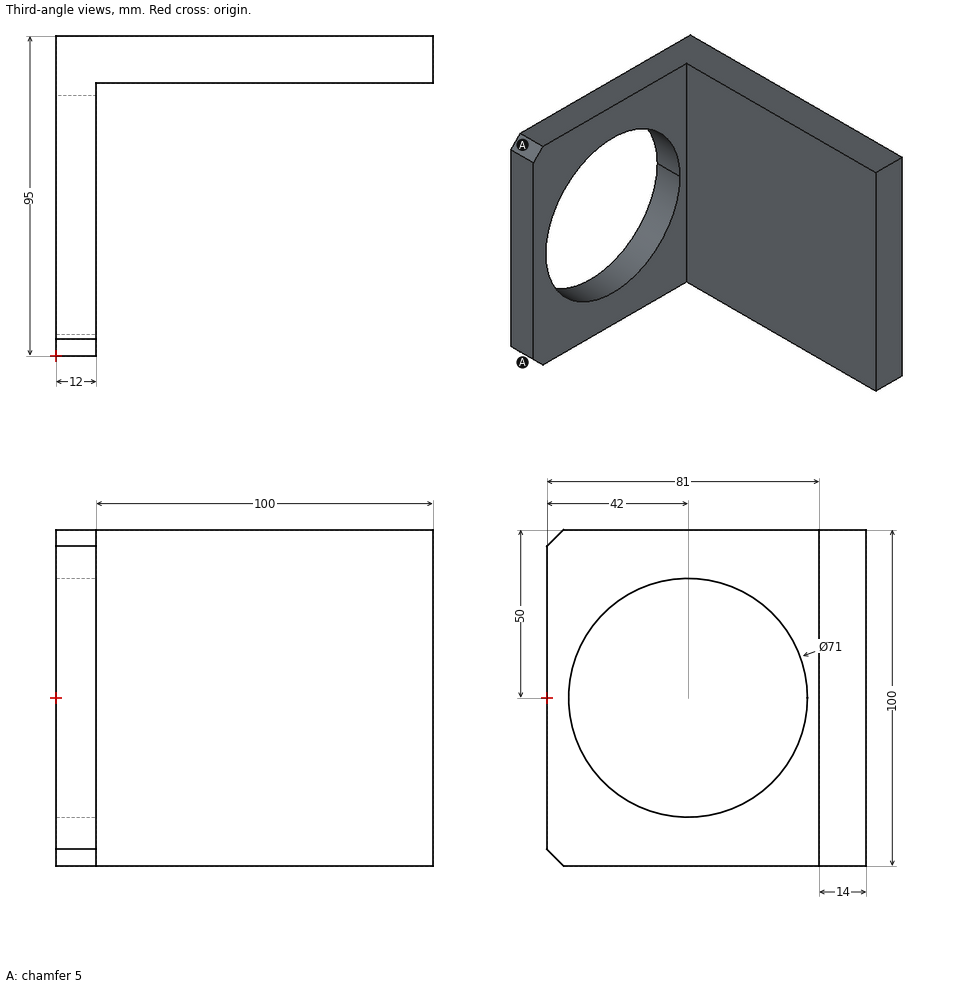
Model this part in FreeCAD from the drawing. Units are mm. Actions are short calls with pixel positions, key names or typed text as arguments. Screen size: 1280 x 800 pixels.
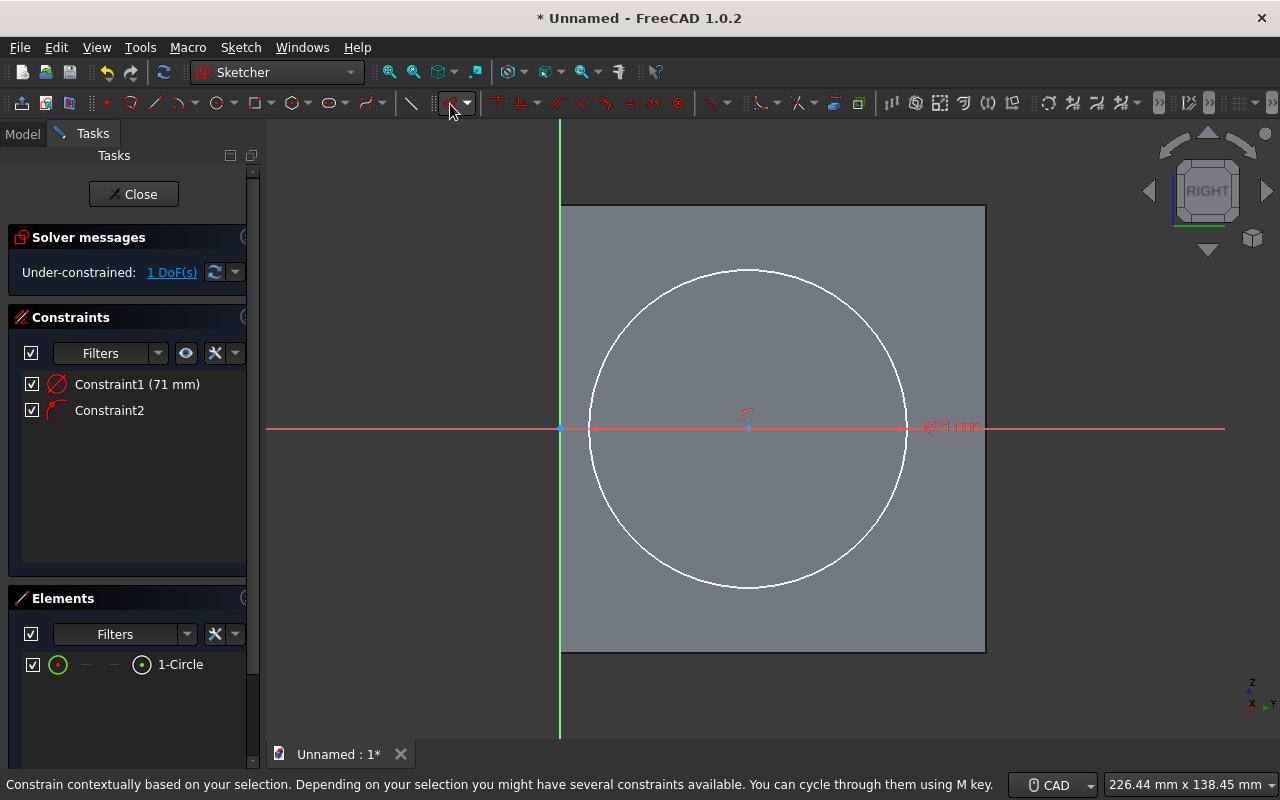
click(748, 429)
click(654, 463)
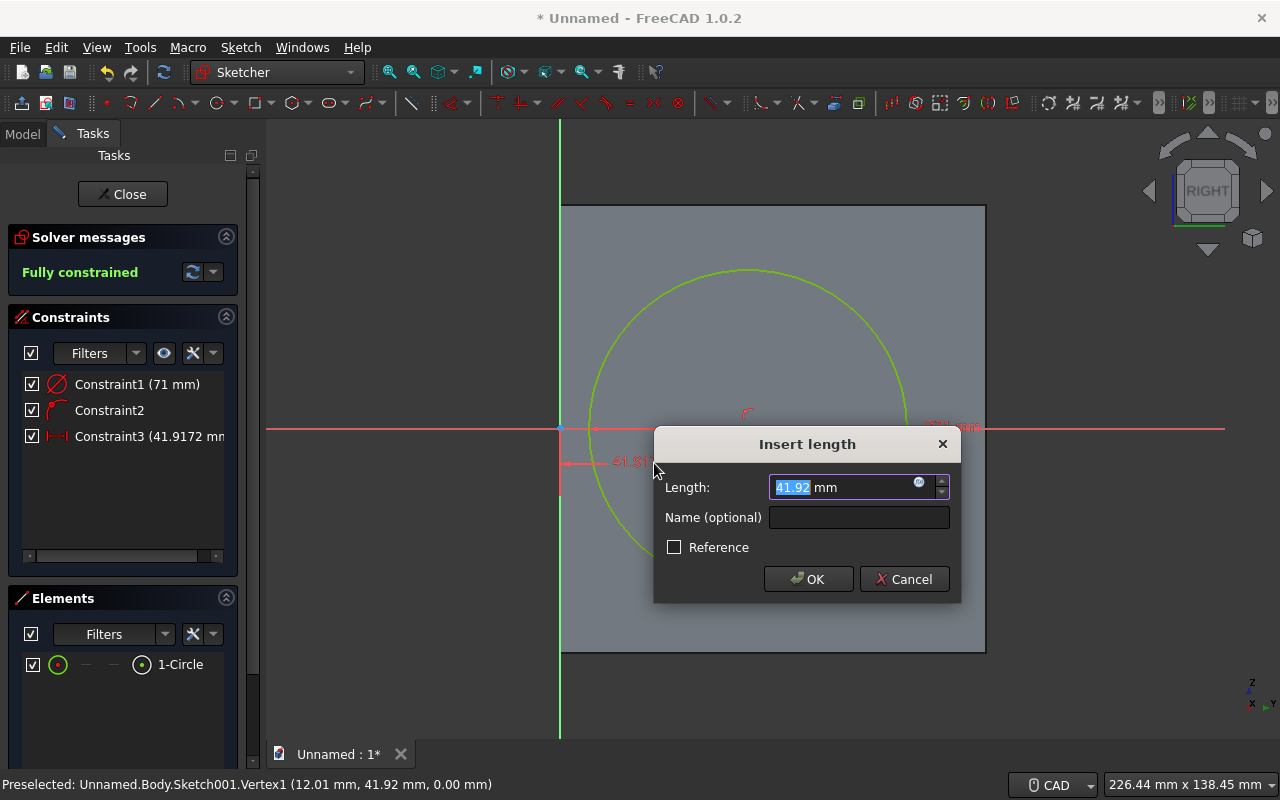
text(42)
key(Return)
key(Escape)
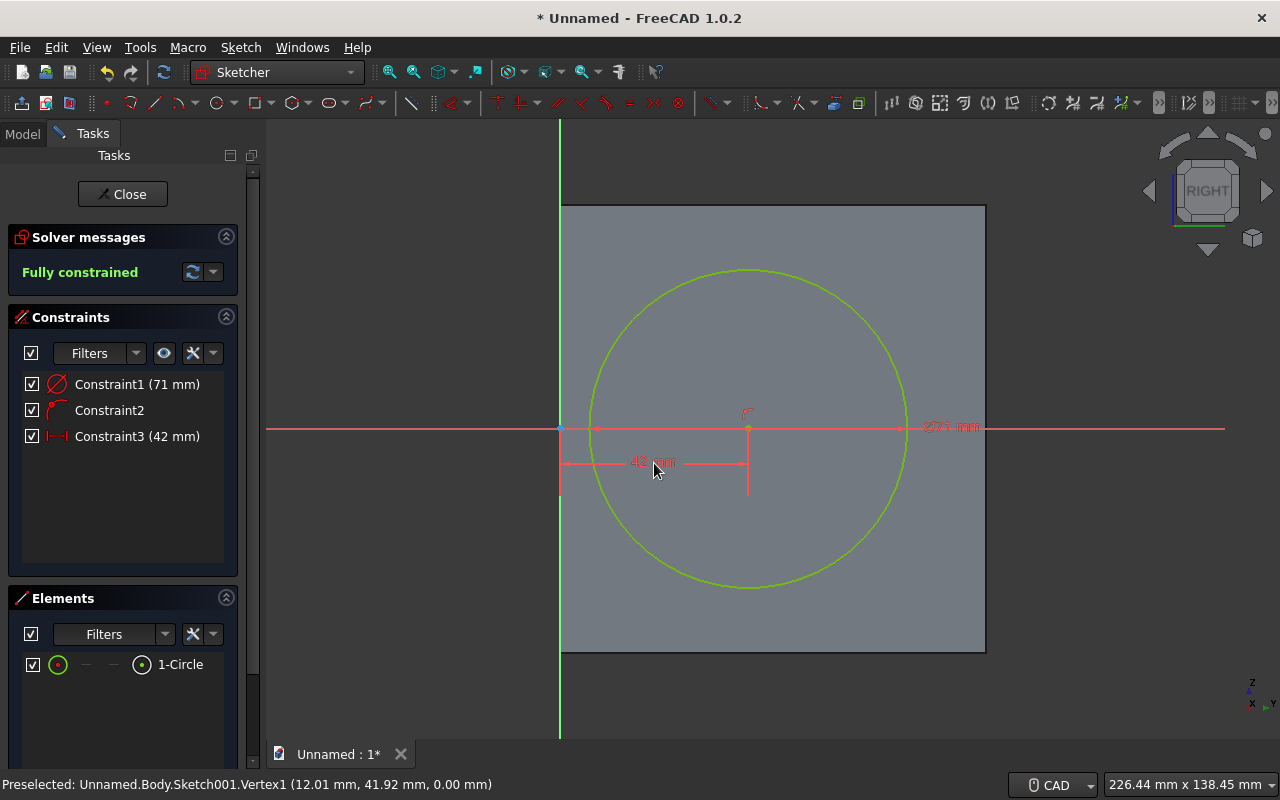
click(123, 194)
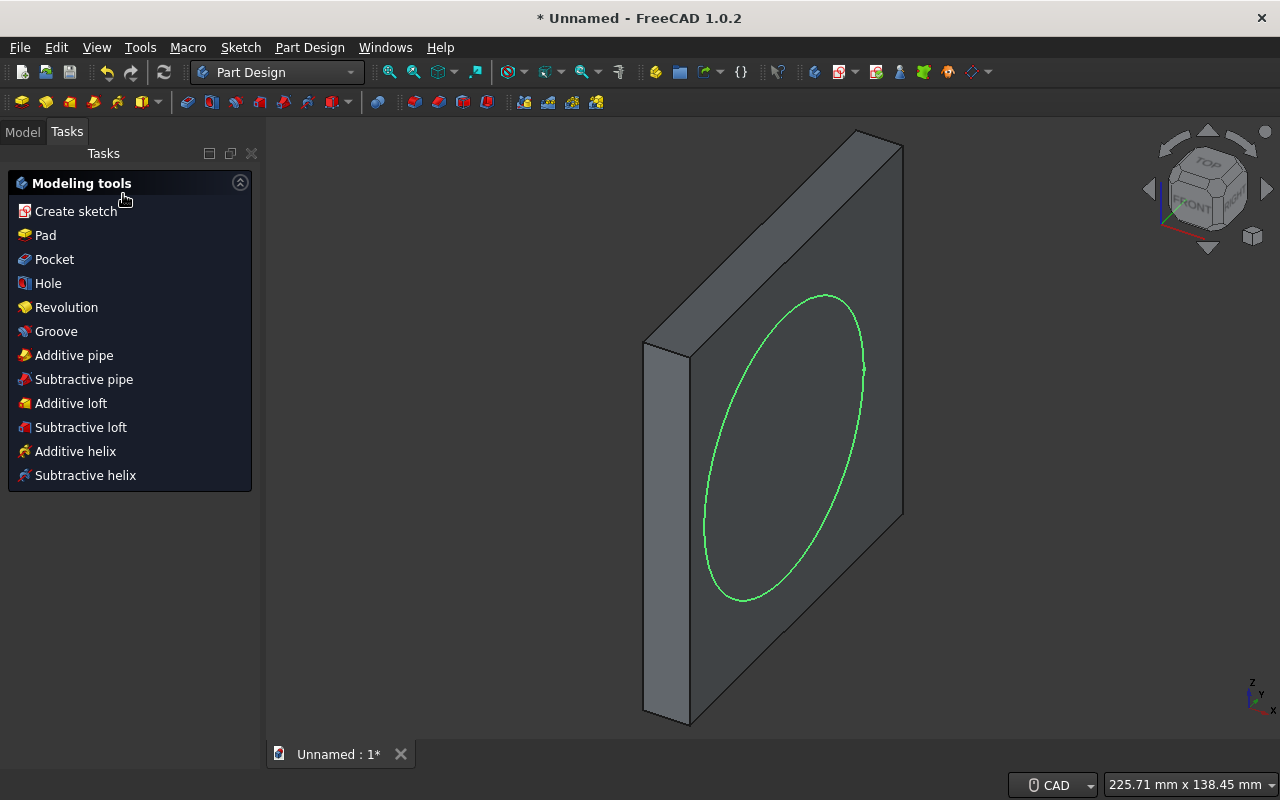
click(188, 102)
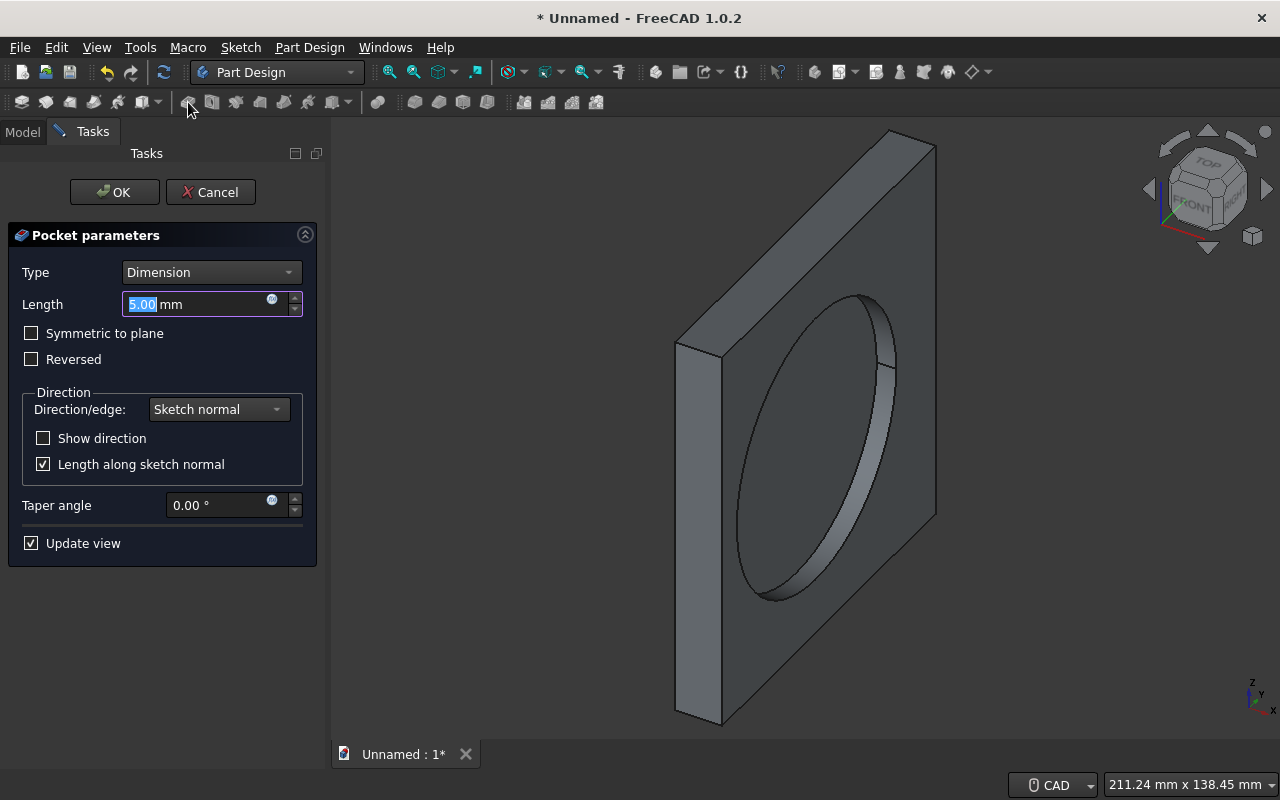
click(212, 272)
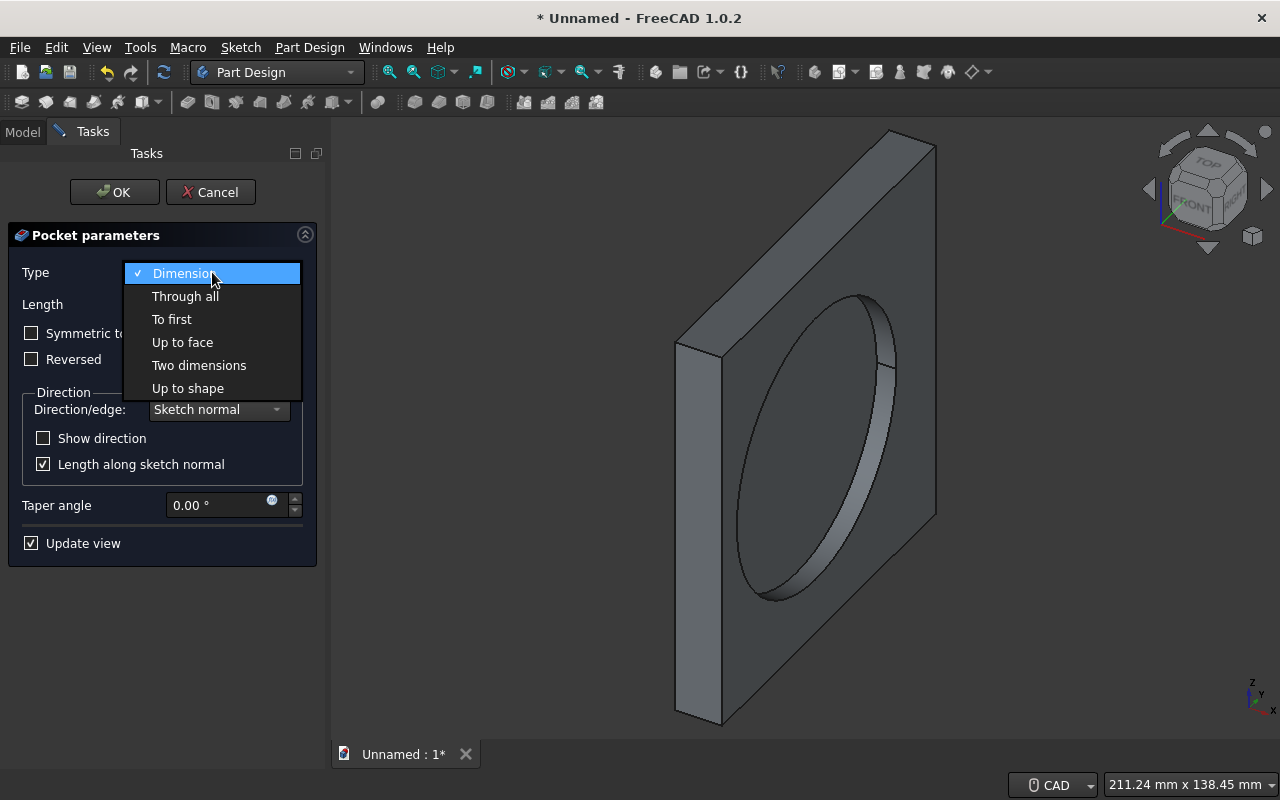
click(212, 320)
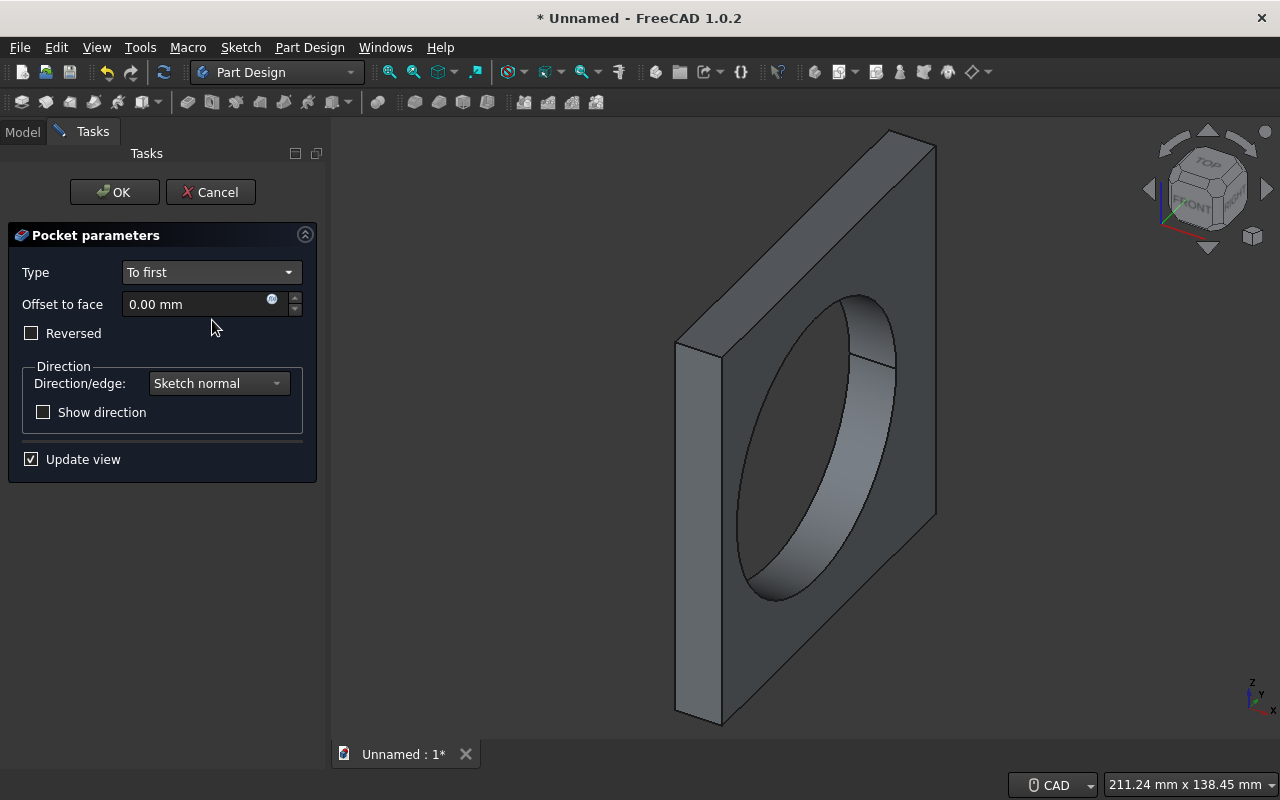
click(115, 192)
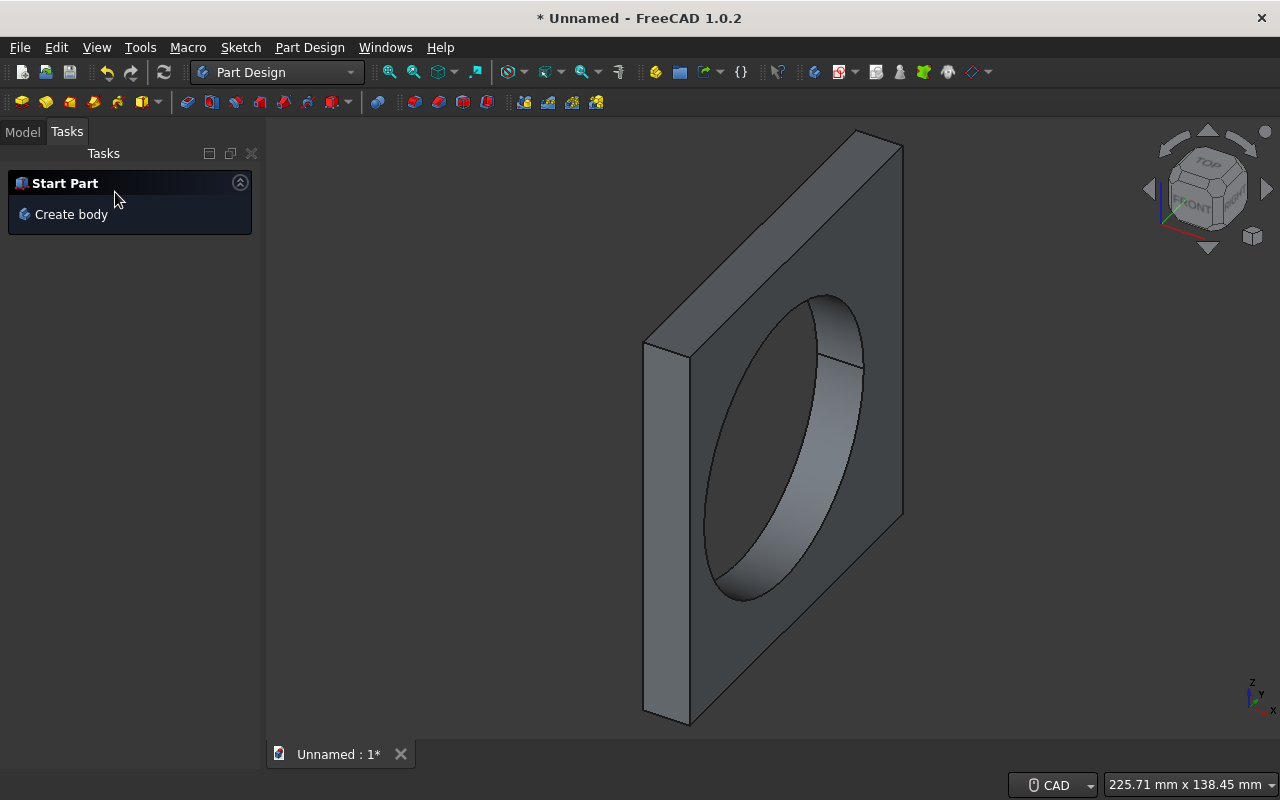
click(857, 269)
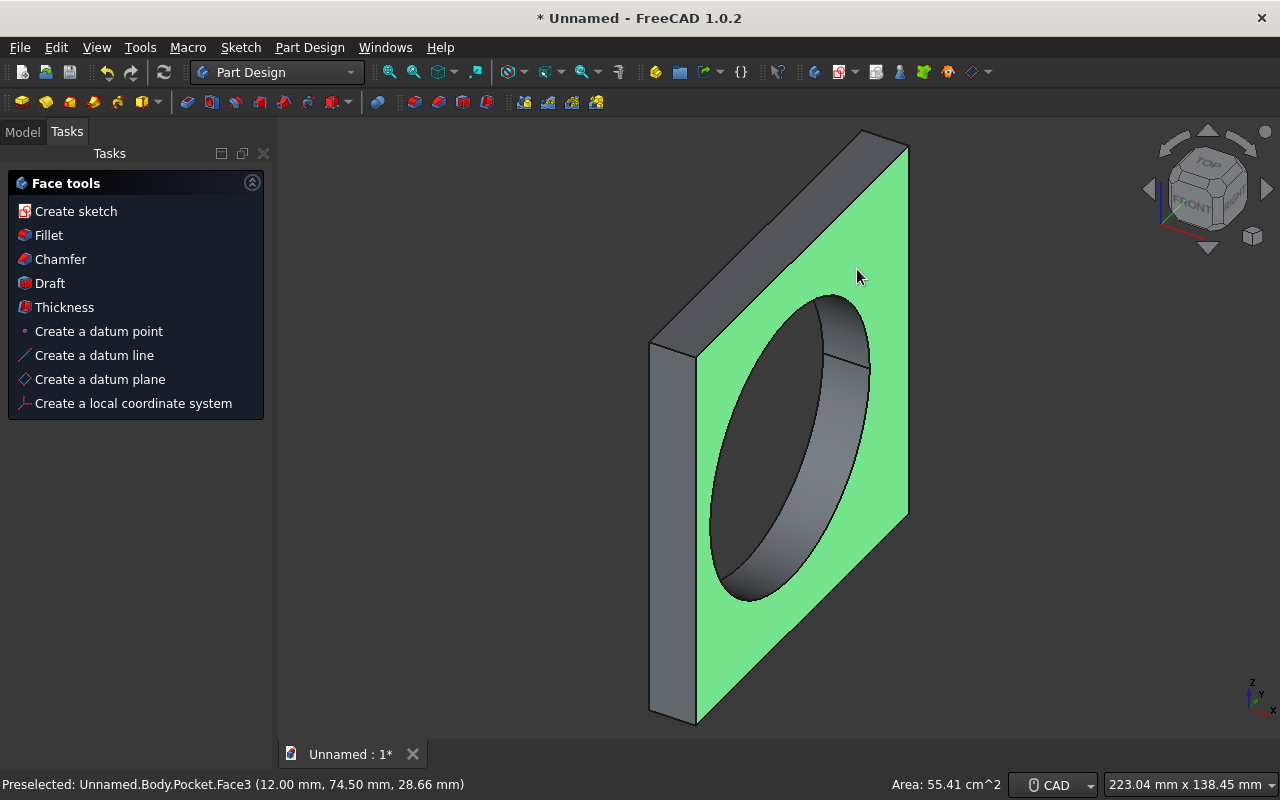
click(840, 72)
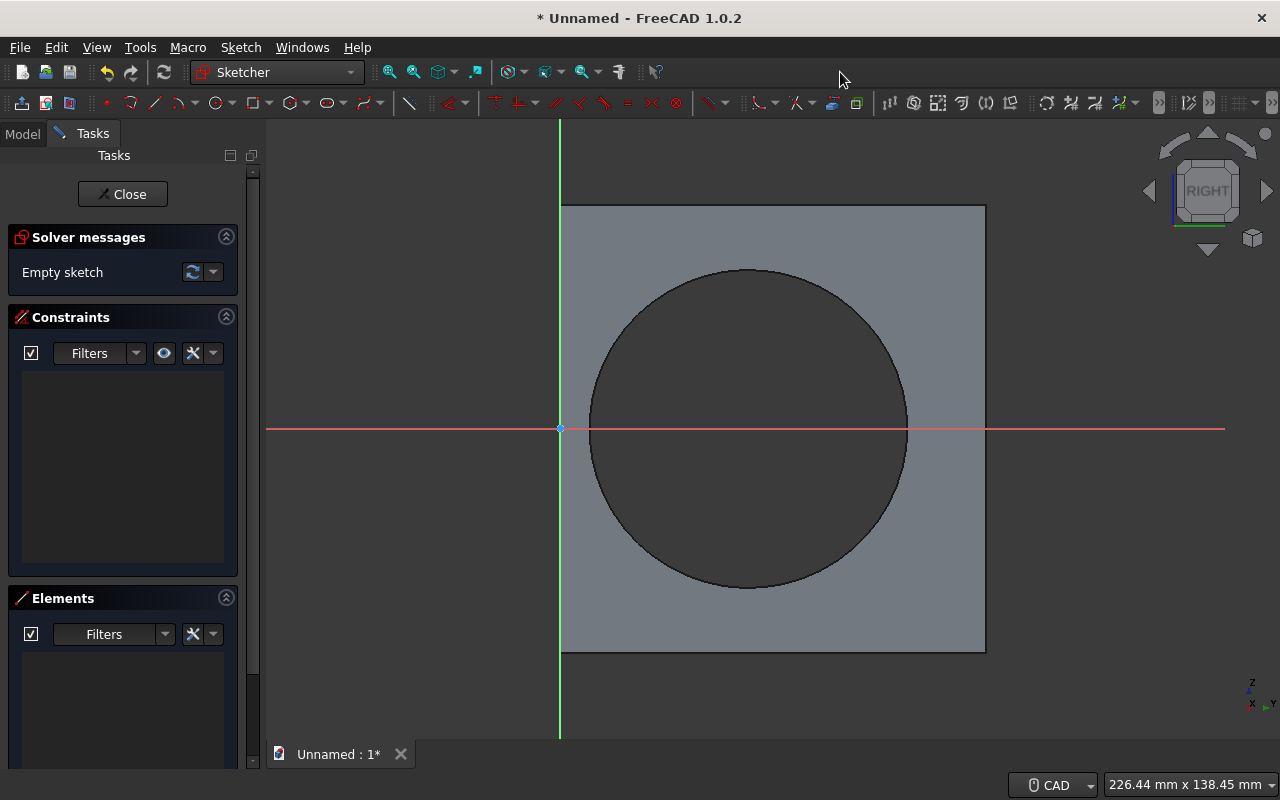
click(254, 104)